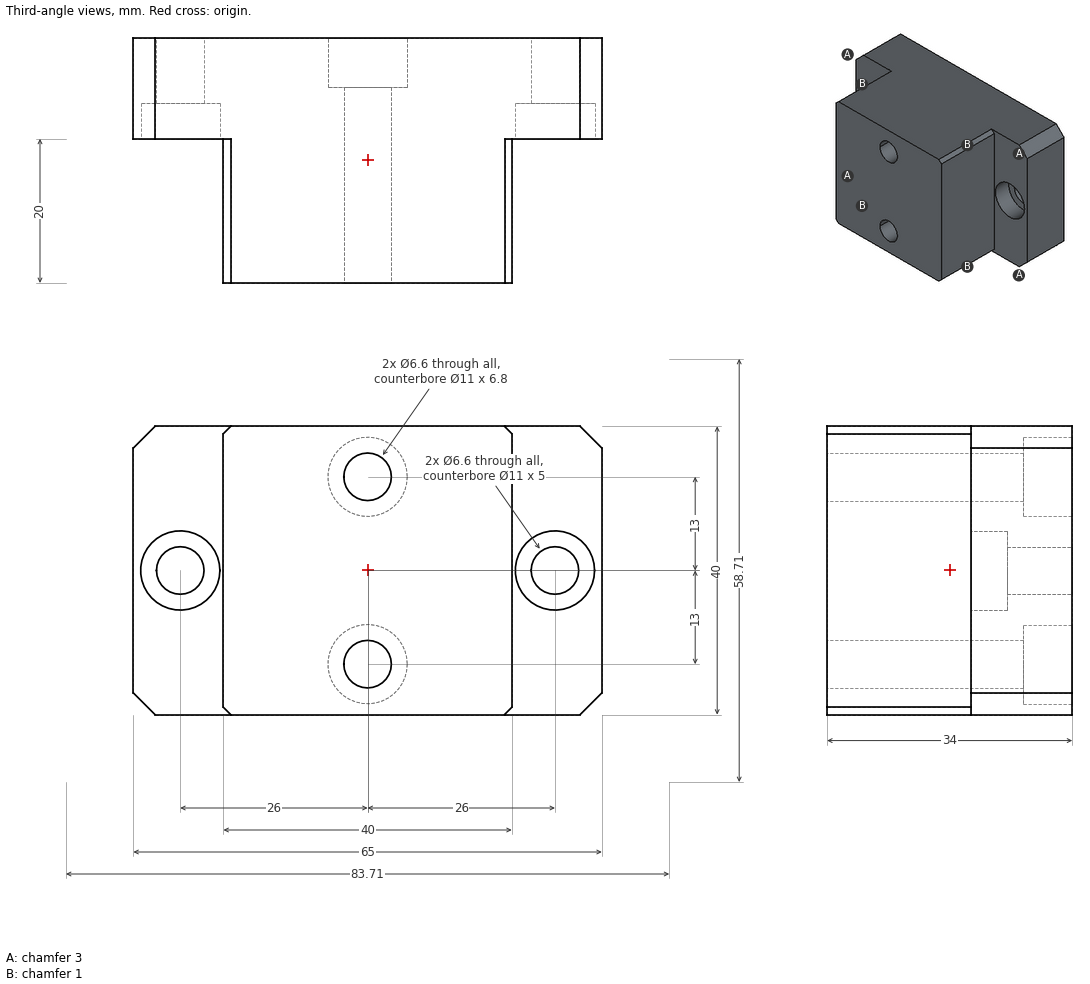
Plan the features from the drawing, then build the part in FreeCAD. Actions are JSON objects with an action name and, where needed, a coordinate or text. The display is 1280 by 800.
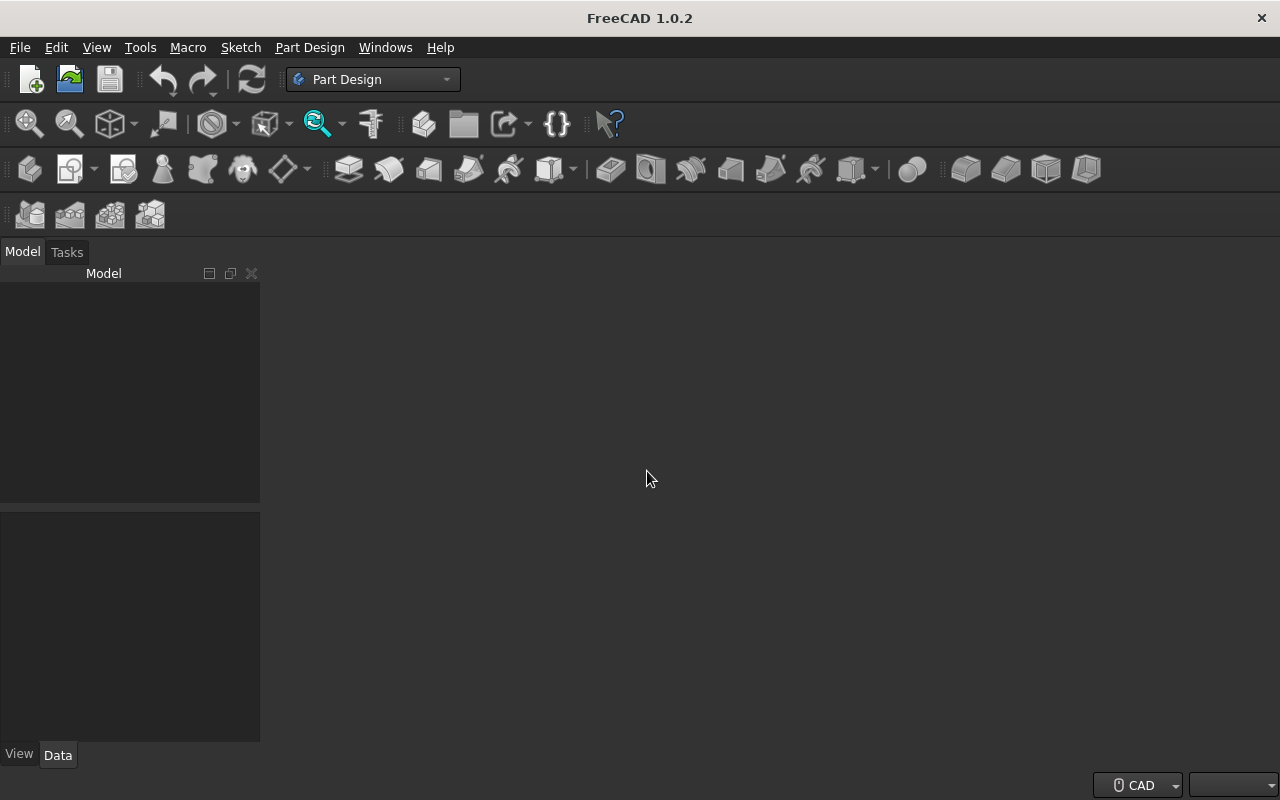
{"action": "left_click", "coordinate": [30, 80]}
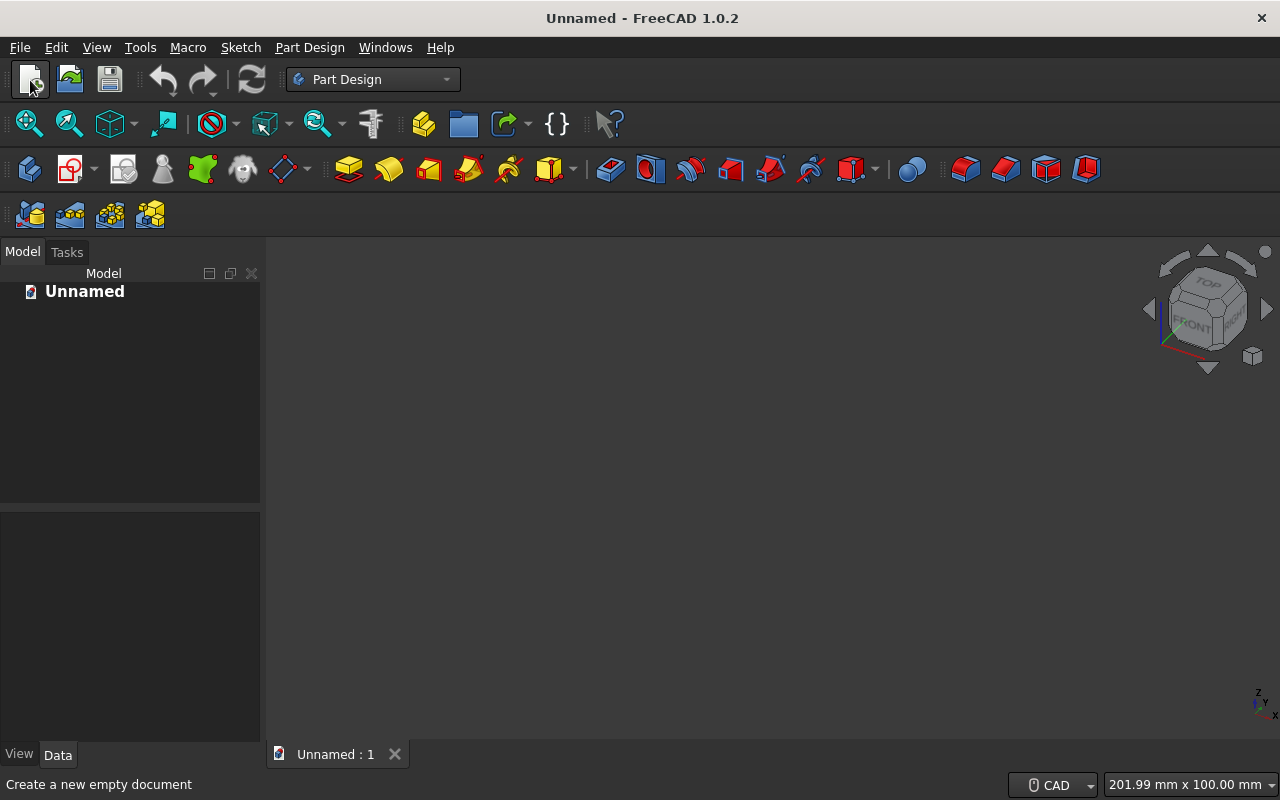
{"action": "left_click", "coordinate": [70, 170]}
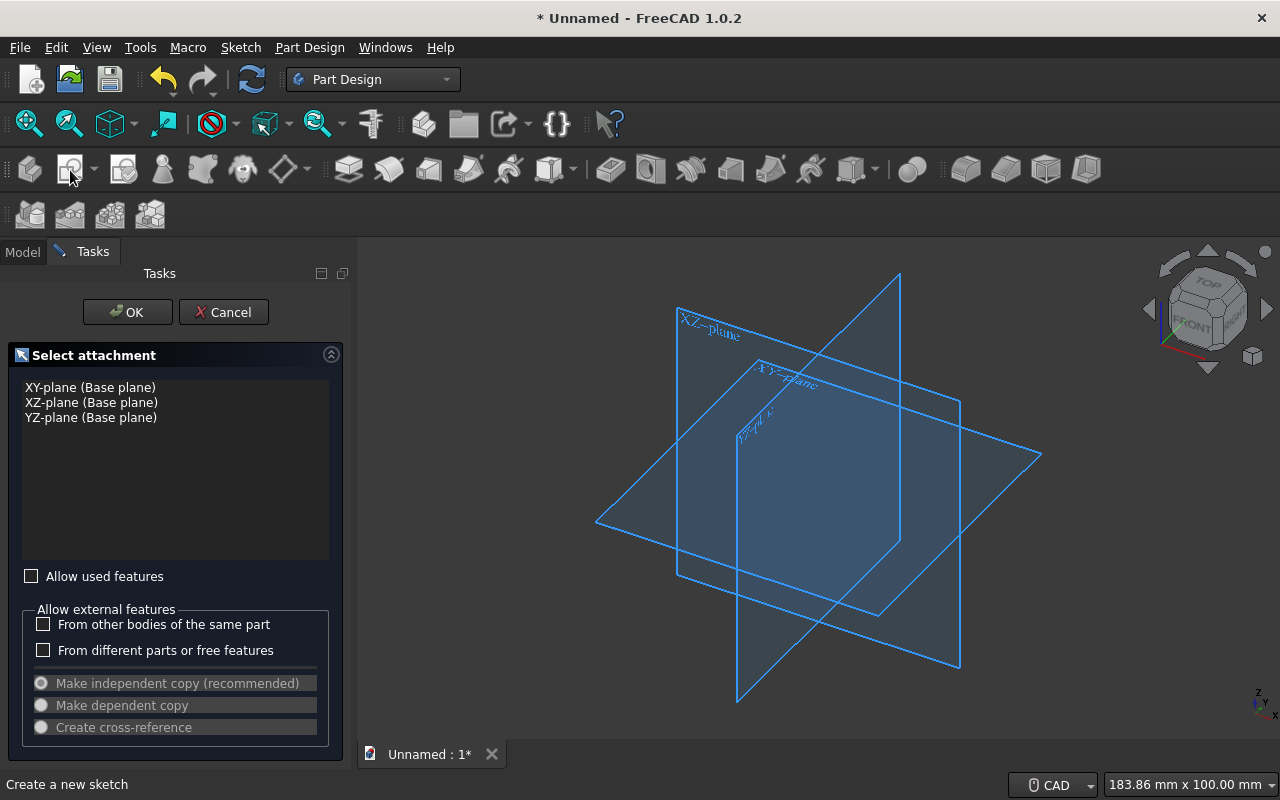
{"action": "left_click", "coordinate": [82, 402]}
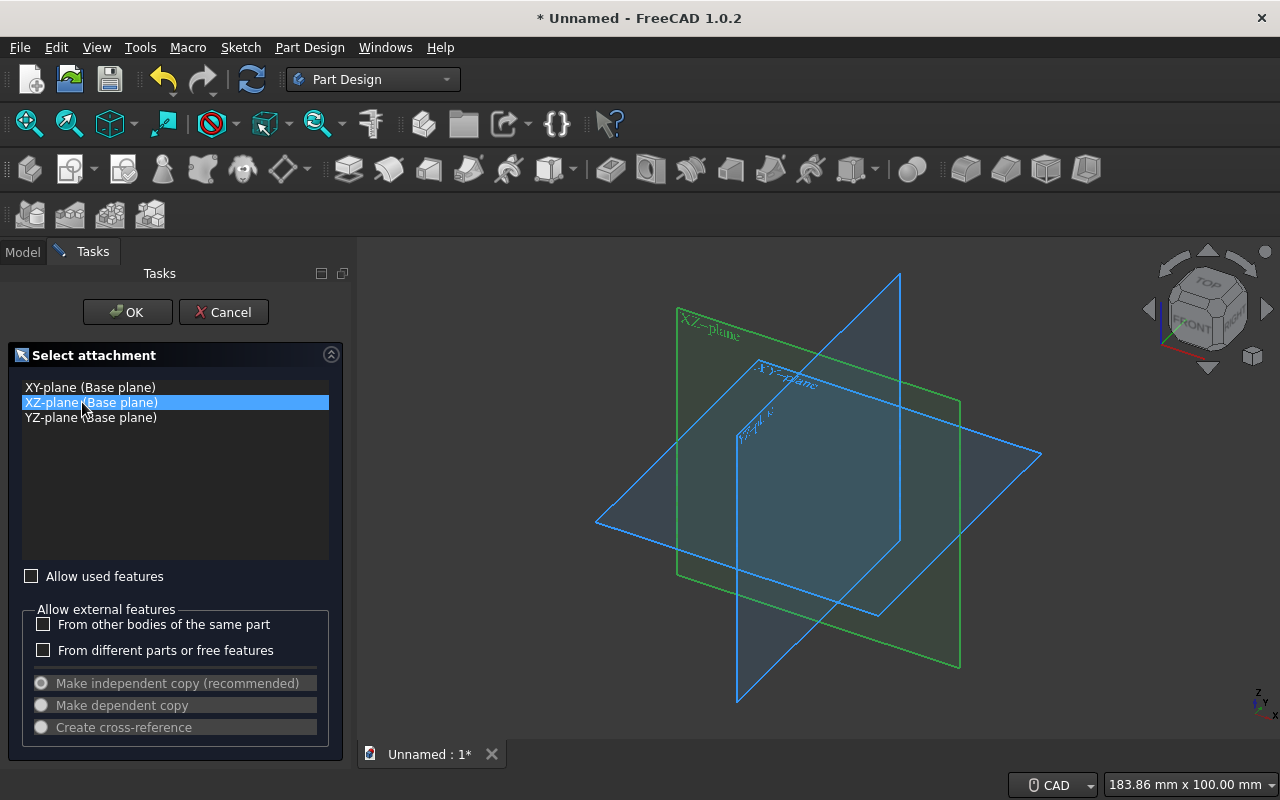
{"action": "left_click", "coordinate": [128, 312]}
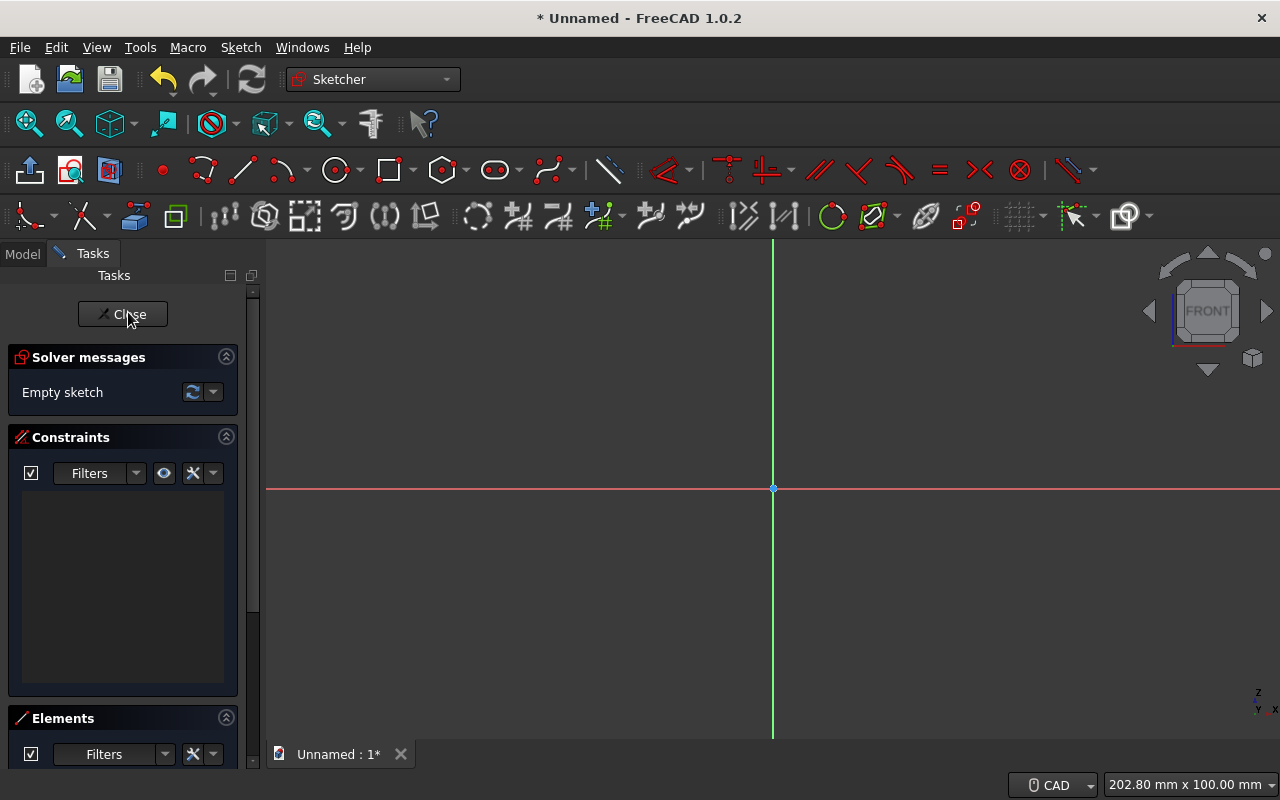
{"action": "scroll", "coordinate": [912, 489], "scroll_direction": "up", "scroll_amount": 2}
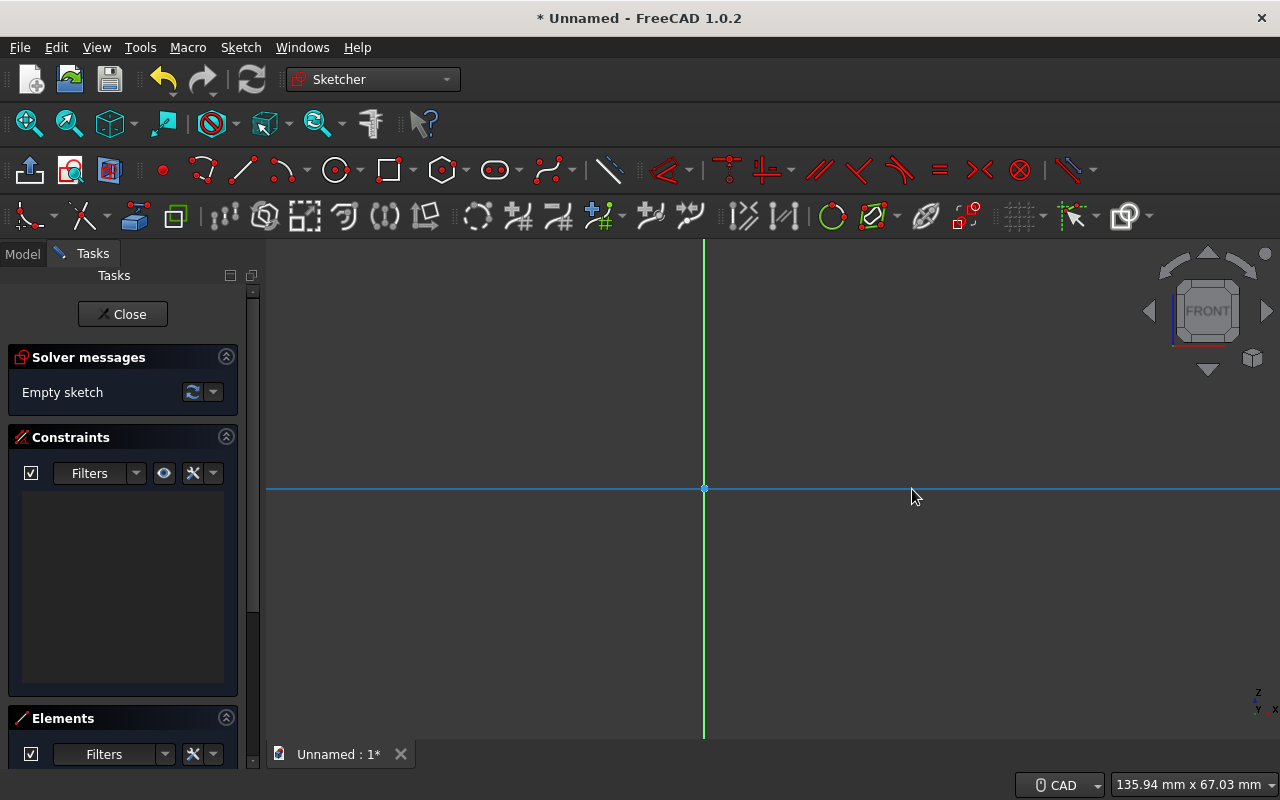
{"action": "left_click", "coordinate": [416, 170]}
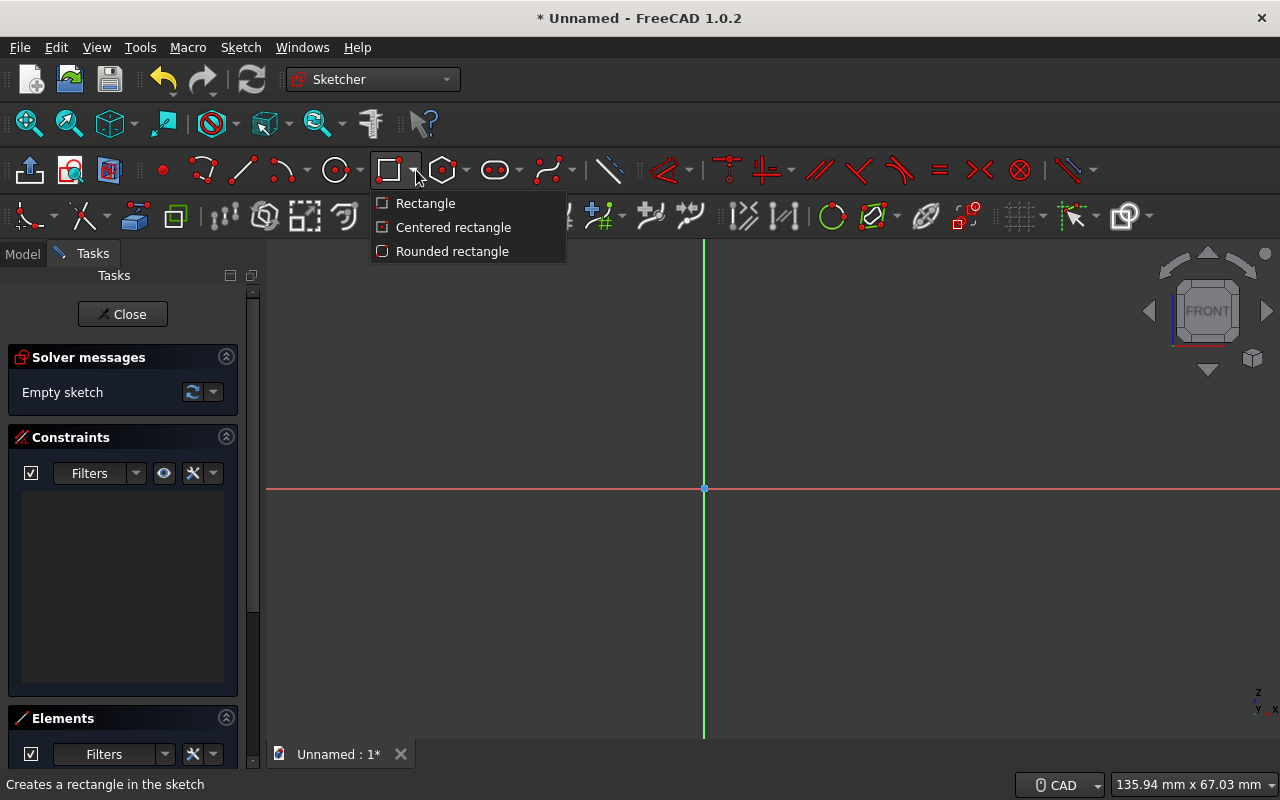
{"action": "left_click", "coordinate": [468, 227]}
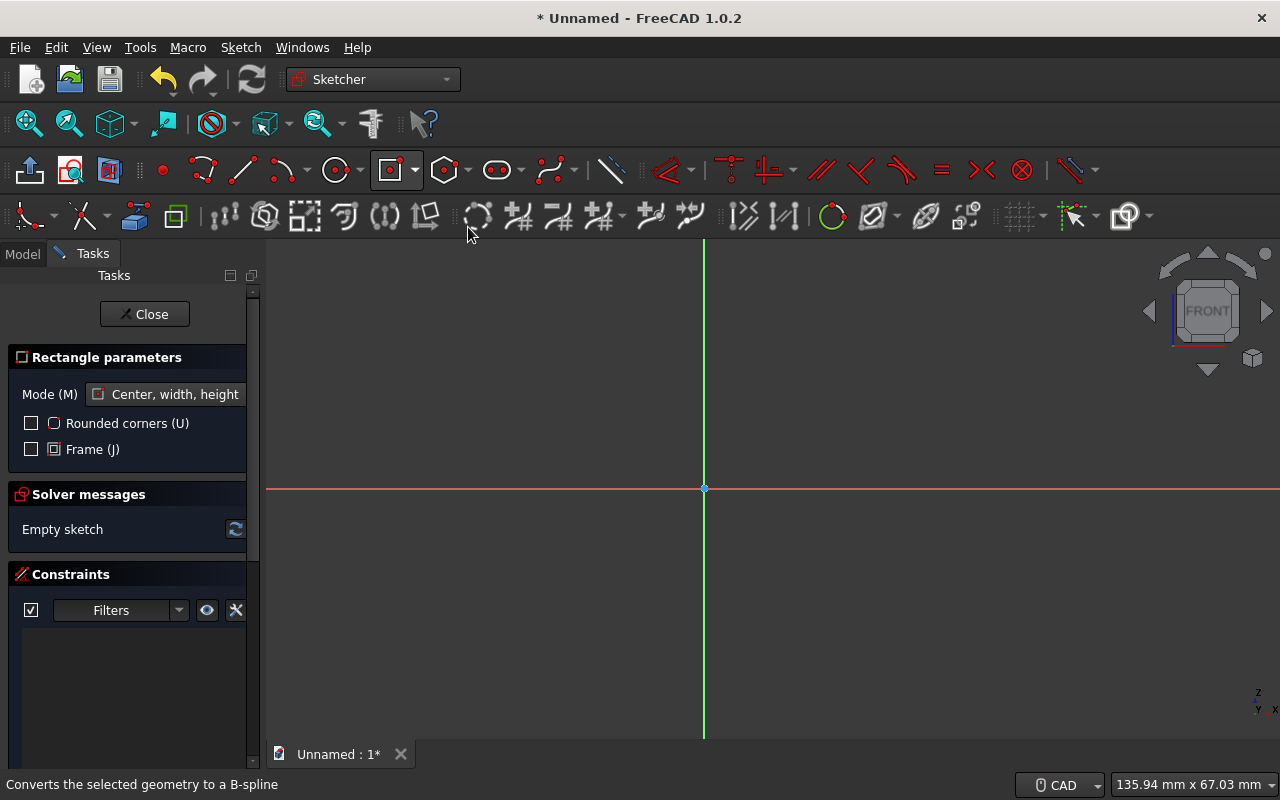
{"action": "left_click", "coordinate": [704, 489]}
{"action": "left_click", "coordinate": [947, 340]}
{"action": "key", "text": "Escape"}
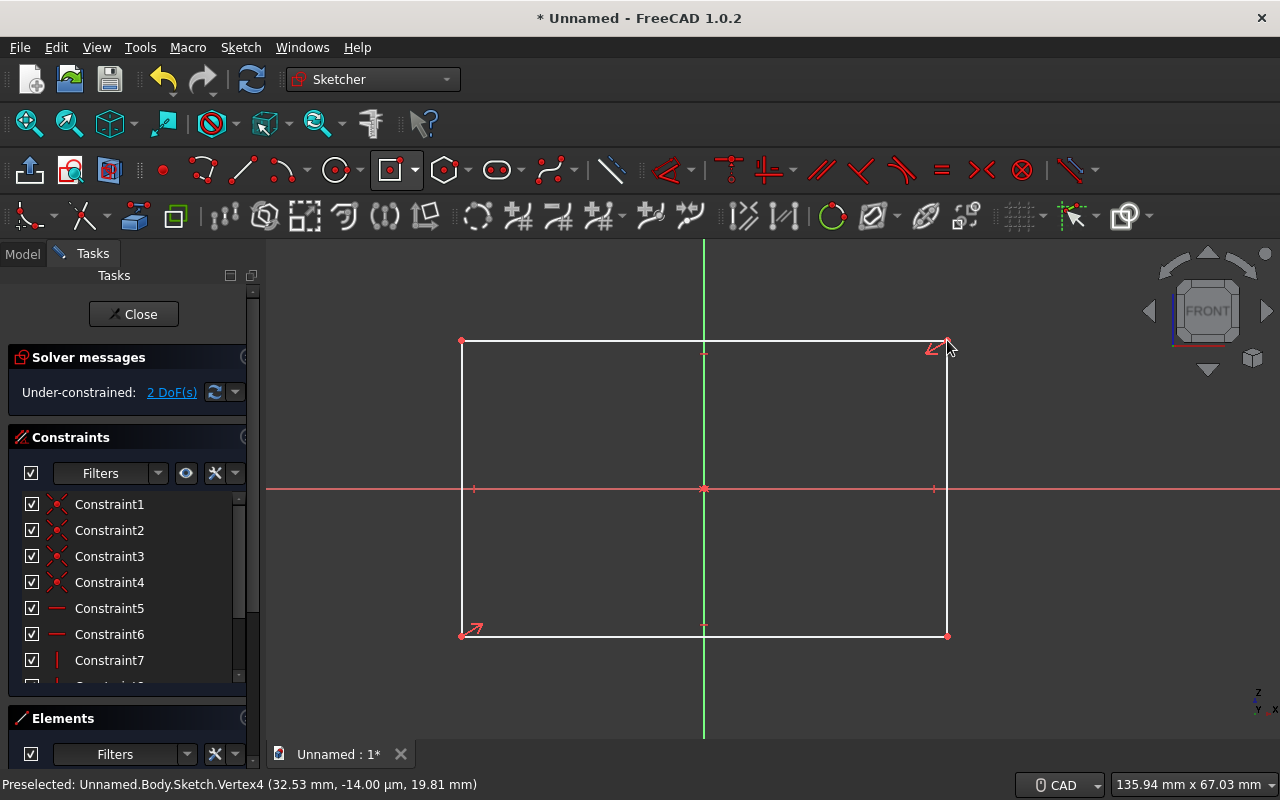
{"action": "left_click", "coordinate": [666, 170]}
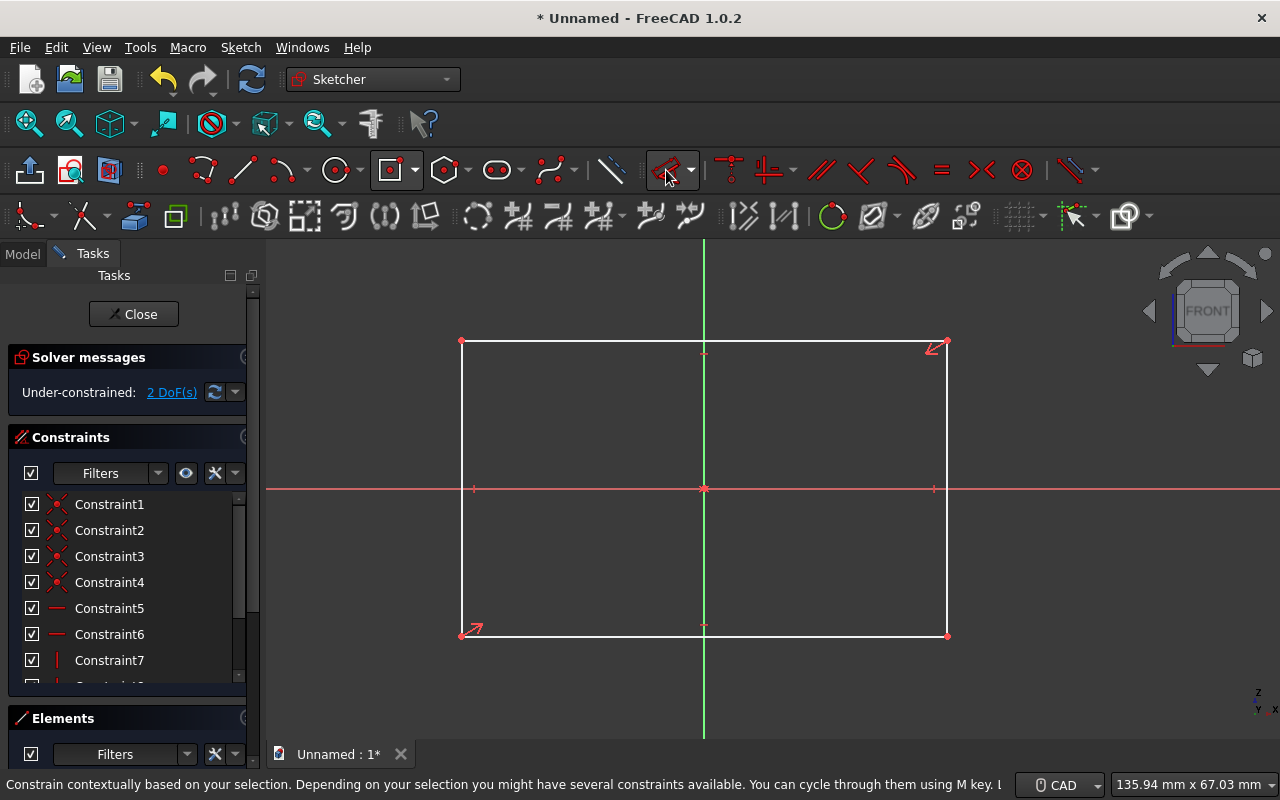
{"action": "left_click", "coordinate": [607, 637]}
{"action": "left_click", "coordinate": [593, 671]}